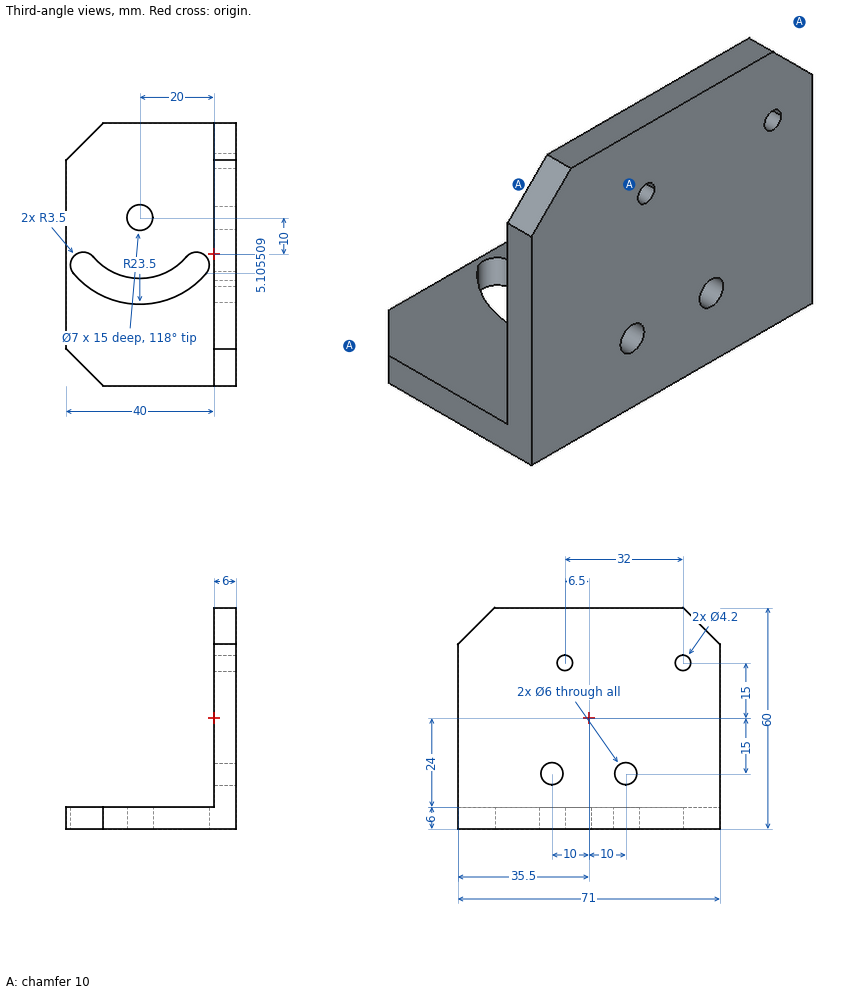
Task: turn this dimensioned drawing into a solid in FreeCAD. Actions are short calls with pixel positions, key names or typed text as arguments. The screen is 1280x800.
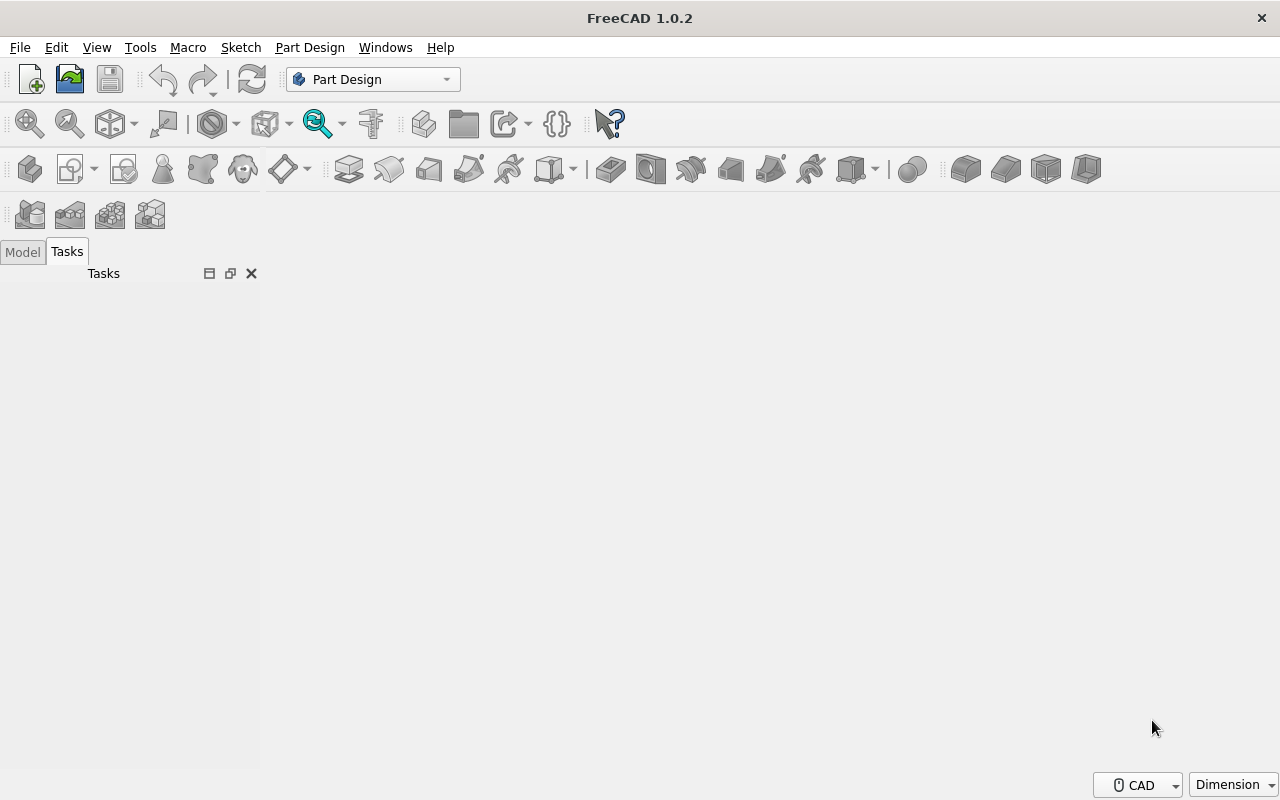
click(1042, 124)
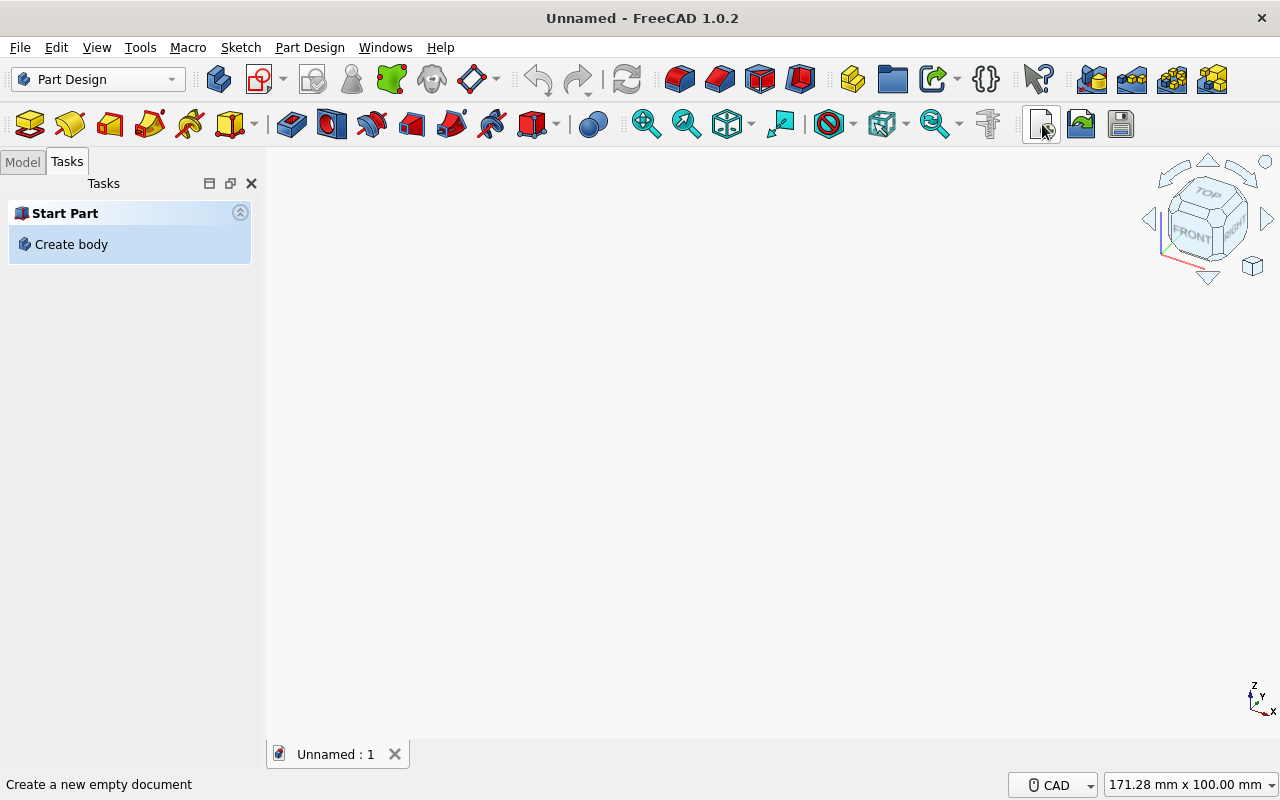
click(260, 80)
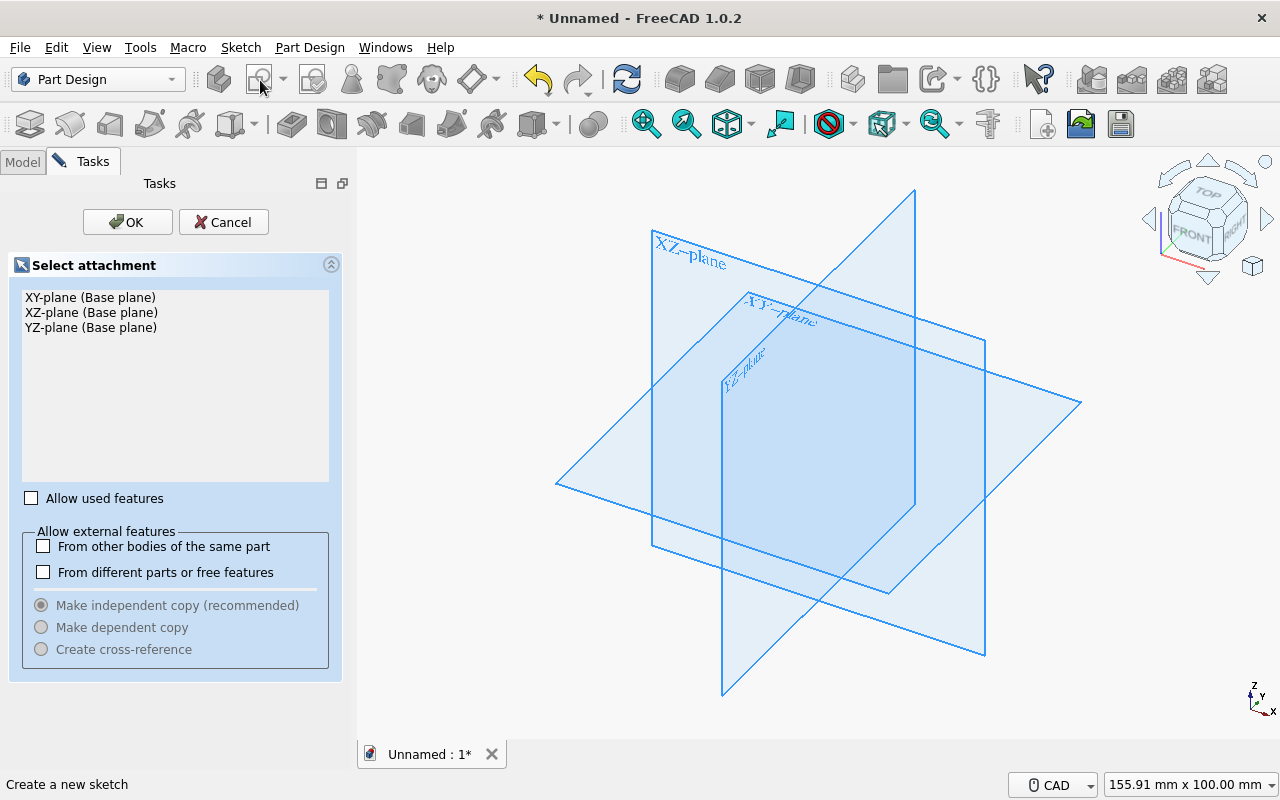
click(82, 328)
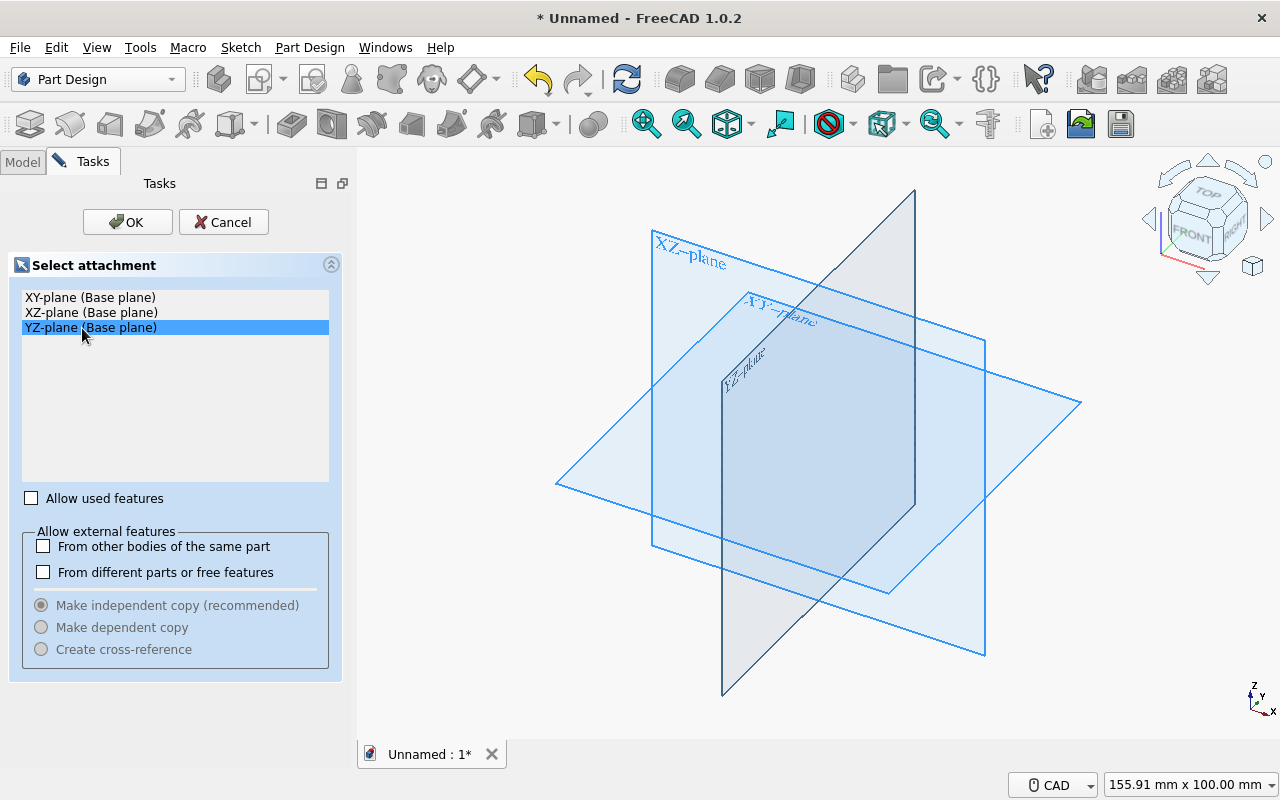
click(128, 222)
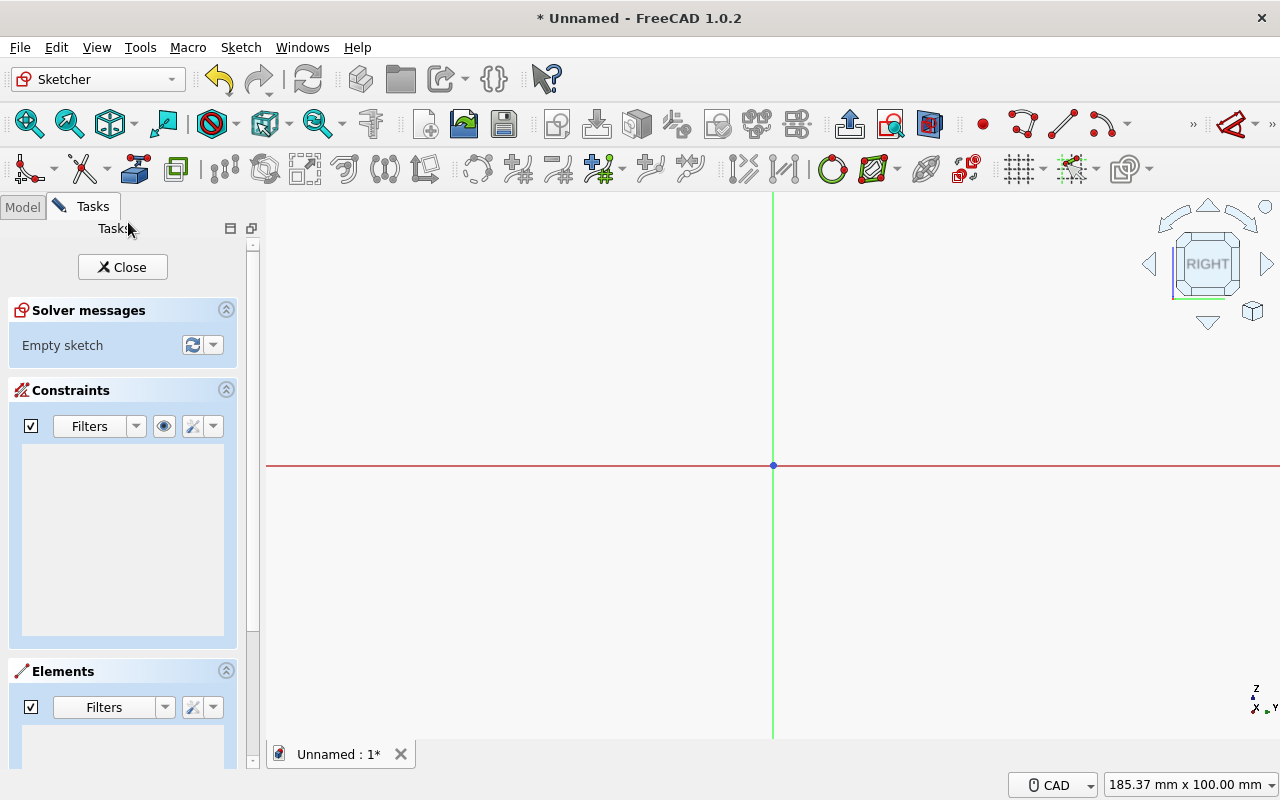
key(g)
key(v)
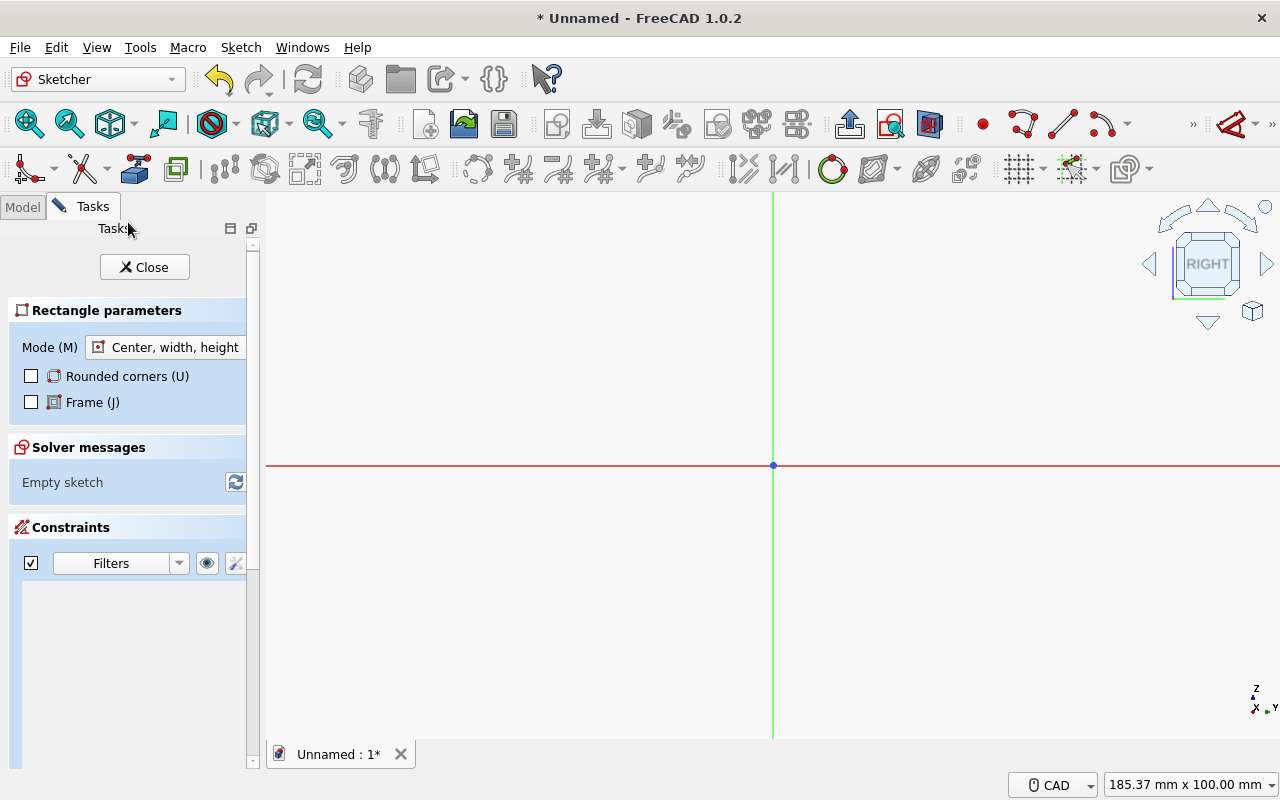
click(773, 466)
click(967, 301)
key(Escape)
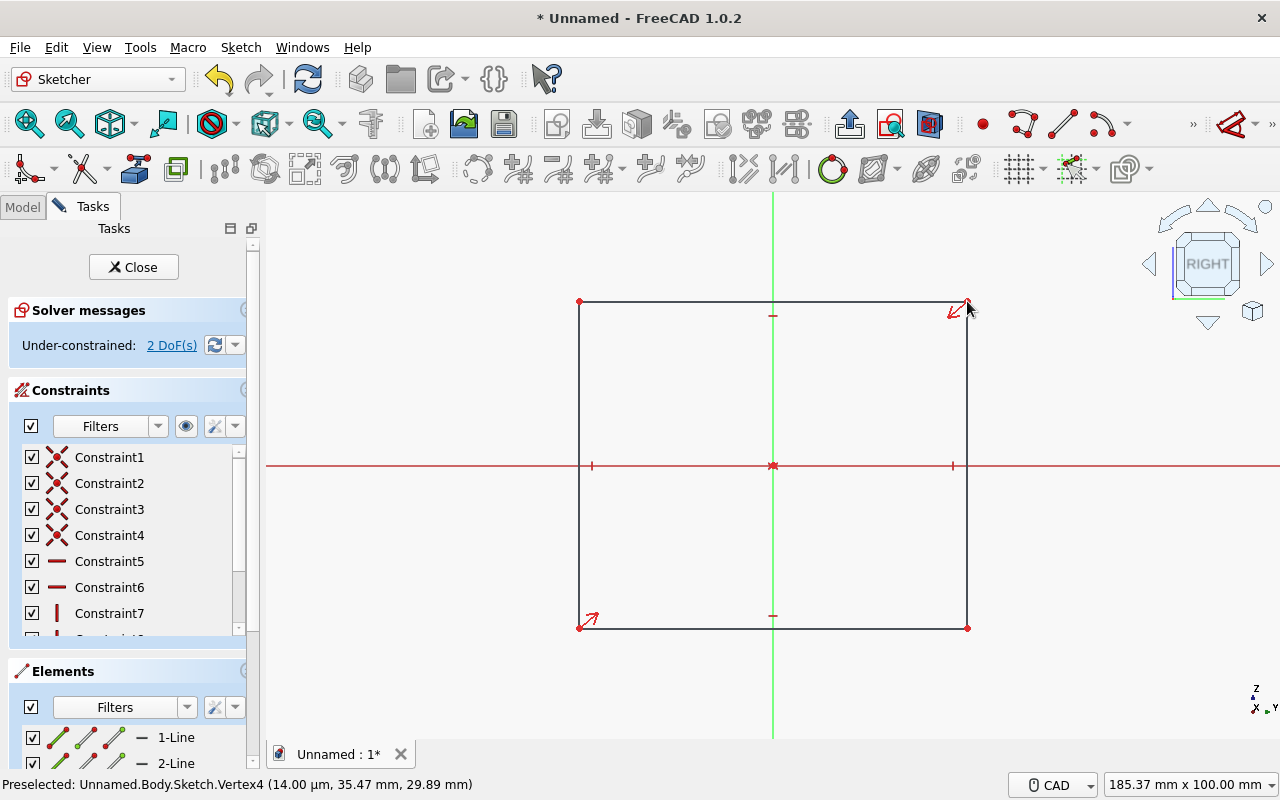
click(1232, 124)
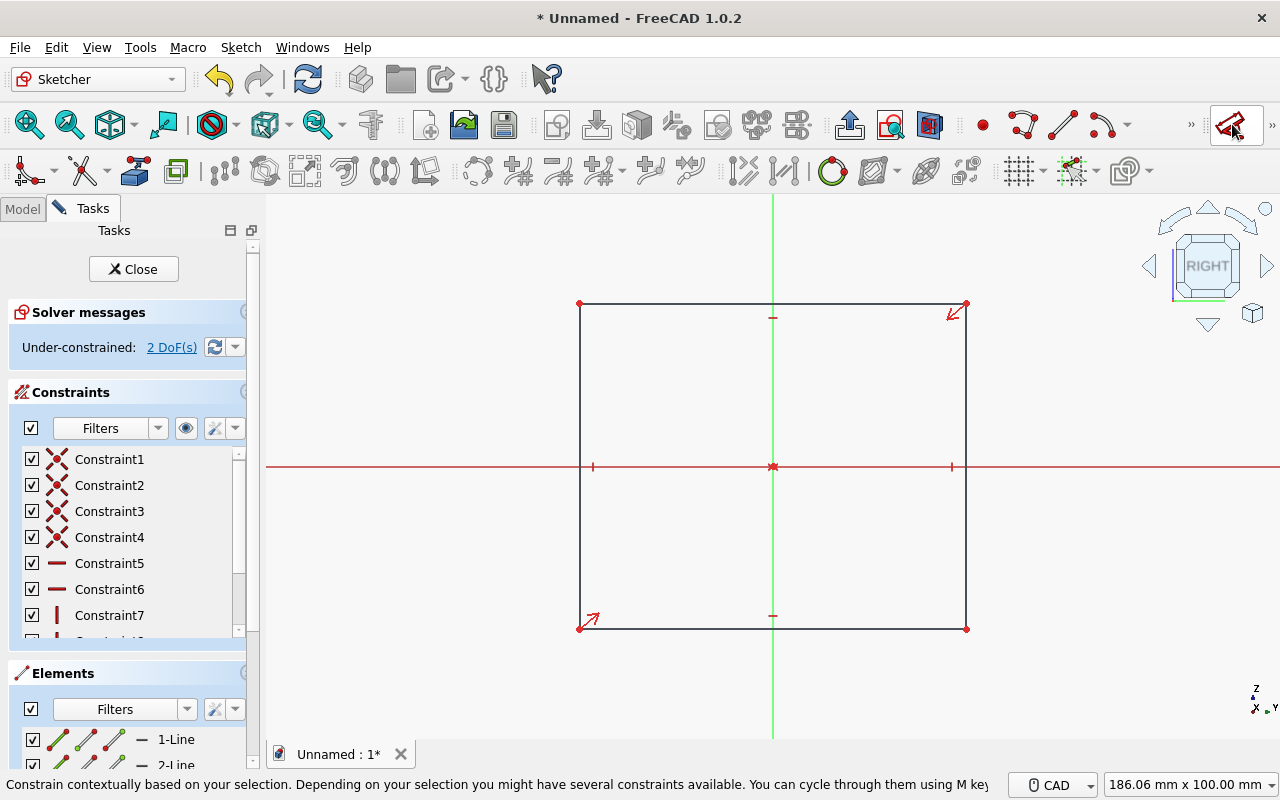
click(696, 629)
click(684, 663)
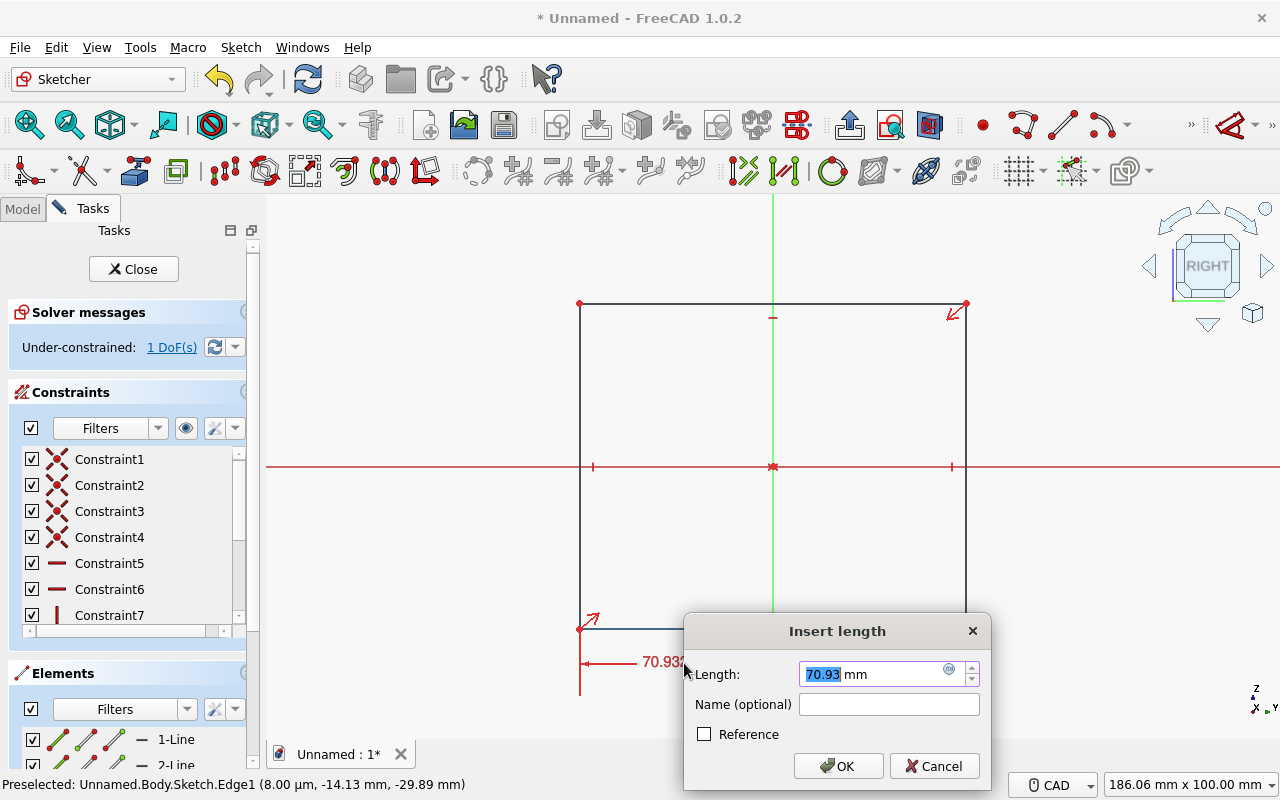
text(71)
key(Return)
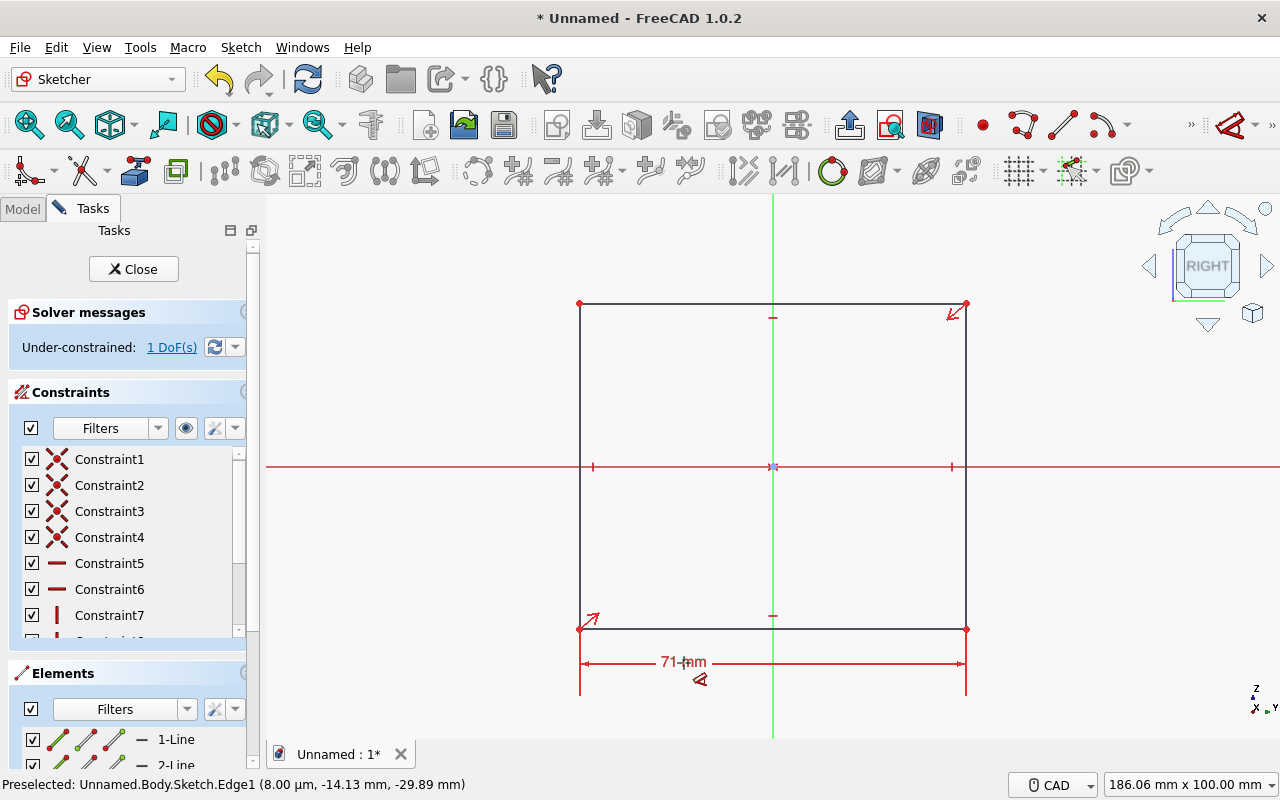
click(966, 532)
click(1000, 392)